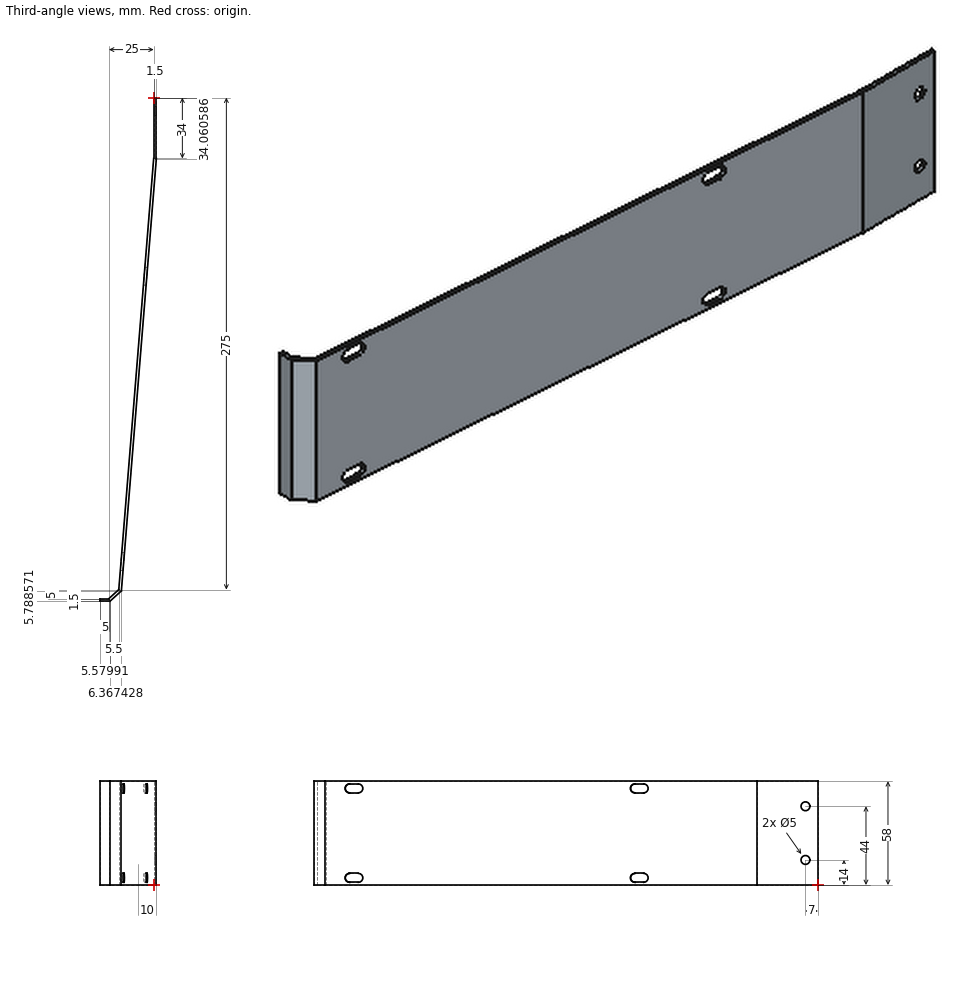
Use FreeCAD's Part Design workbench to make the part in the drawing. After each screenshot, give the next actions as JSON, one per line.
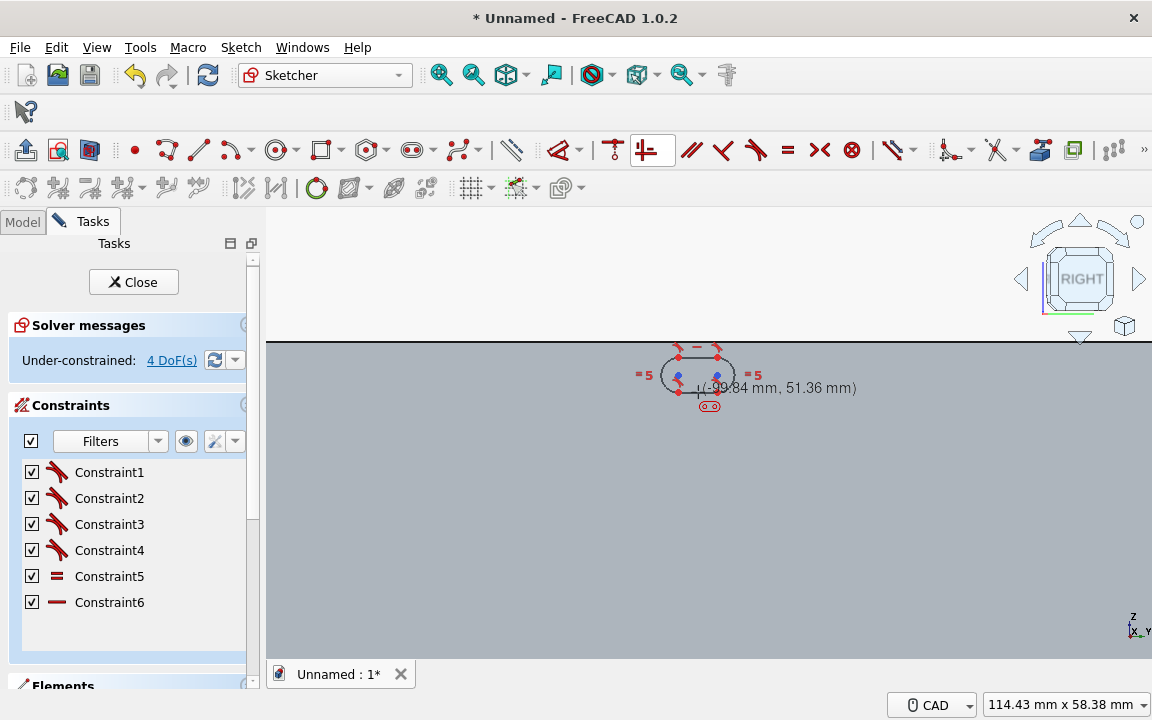
{"action": "scroll", "coordinate": [704, 388], "scroll_direction": "down", "scroll_amount": 7}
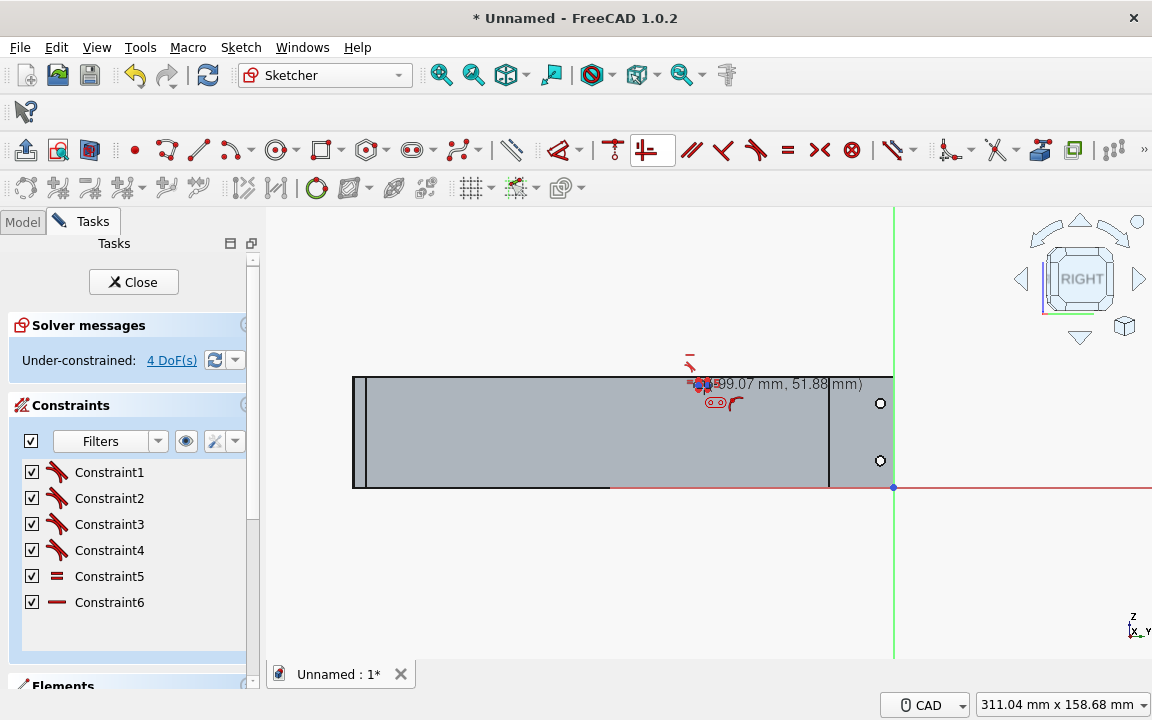
{"action": "scroll", "coordinate": [393, 385], "scroll_direction": "up", "scroll_amount": 8}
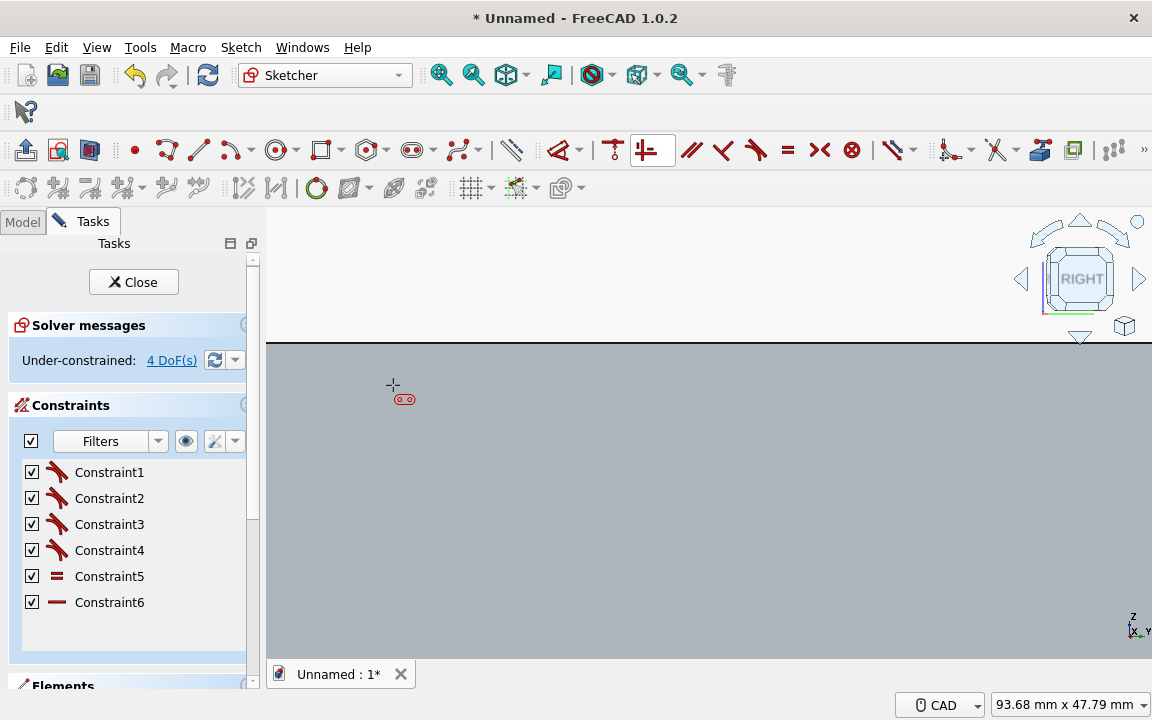
{"action": "scroll", "coordinate": [393, 385], "scroll_direction": "down", "scroll_amount": 8}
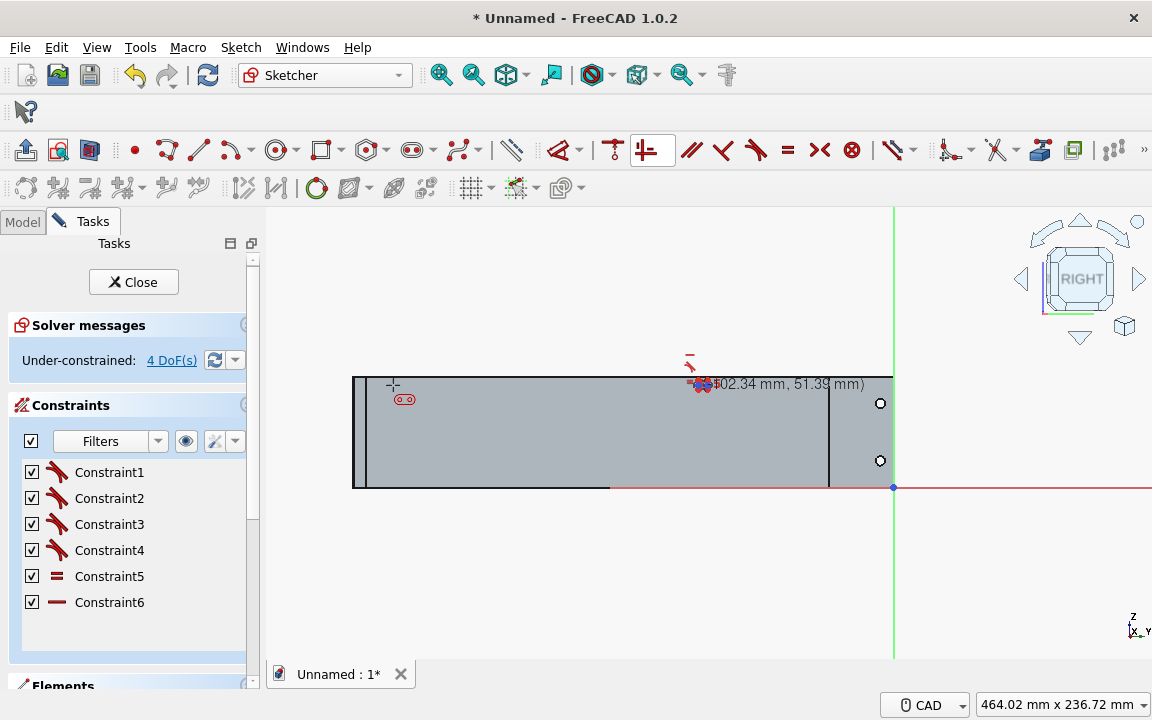
{"action": "left_click", "coordinate": [393, 385]}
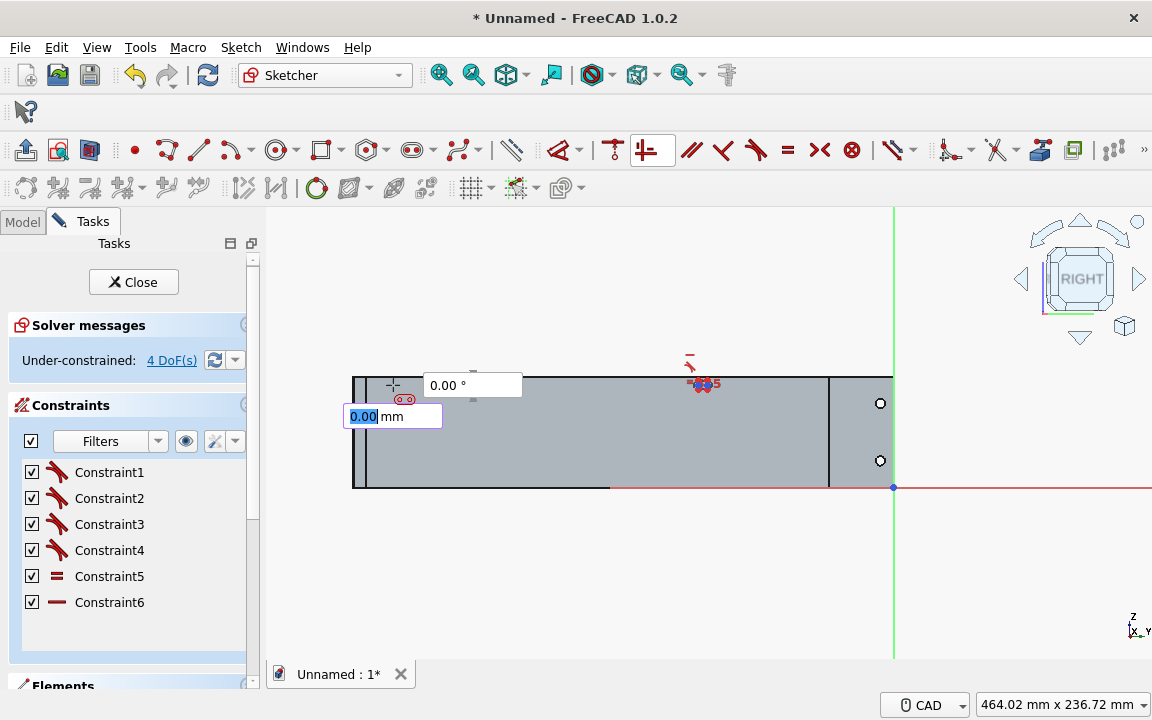
{"action": "scroll", "coordinate": [402, 385], "scroll_direction": "up", "scroll_amount": 3}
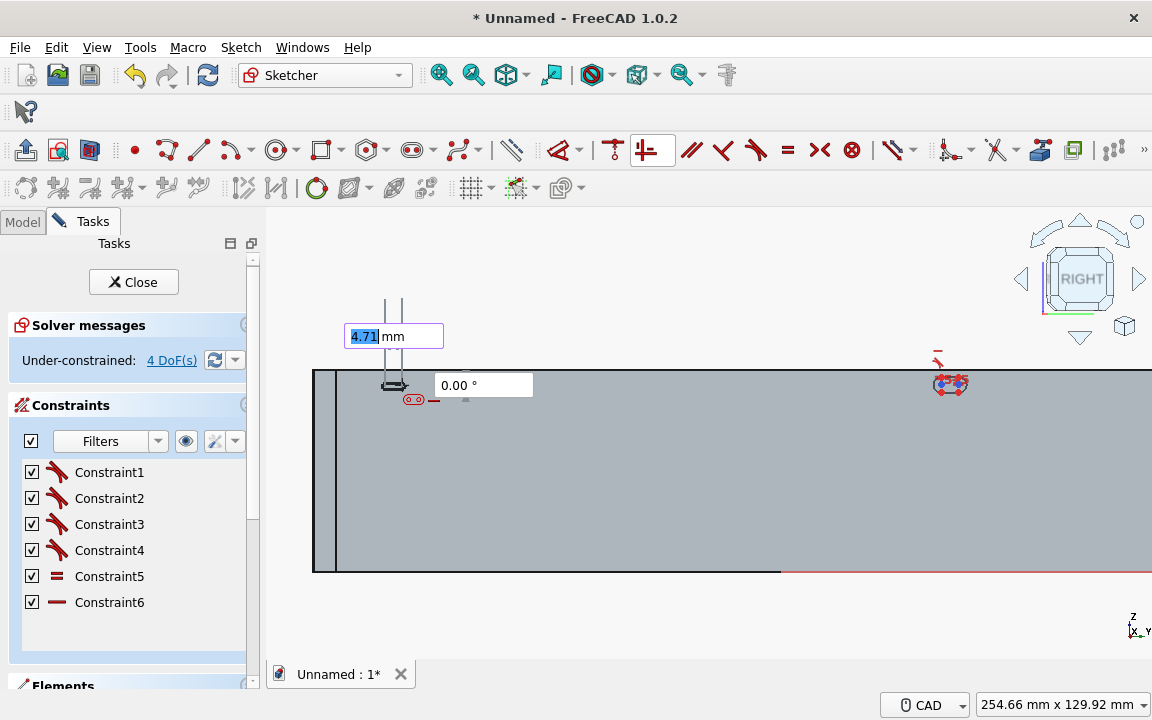
{"action": "left_click", "coordinate": [402, 385]}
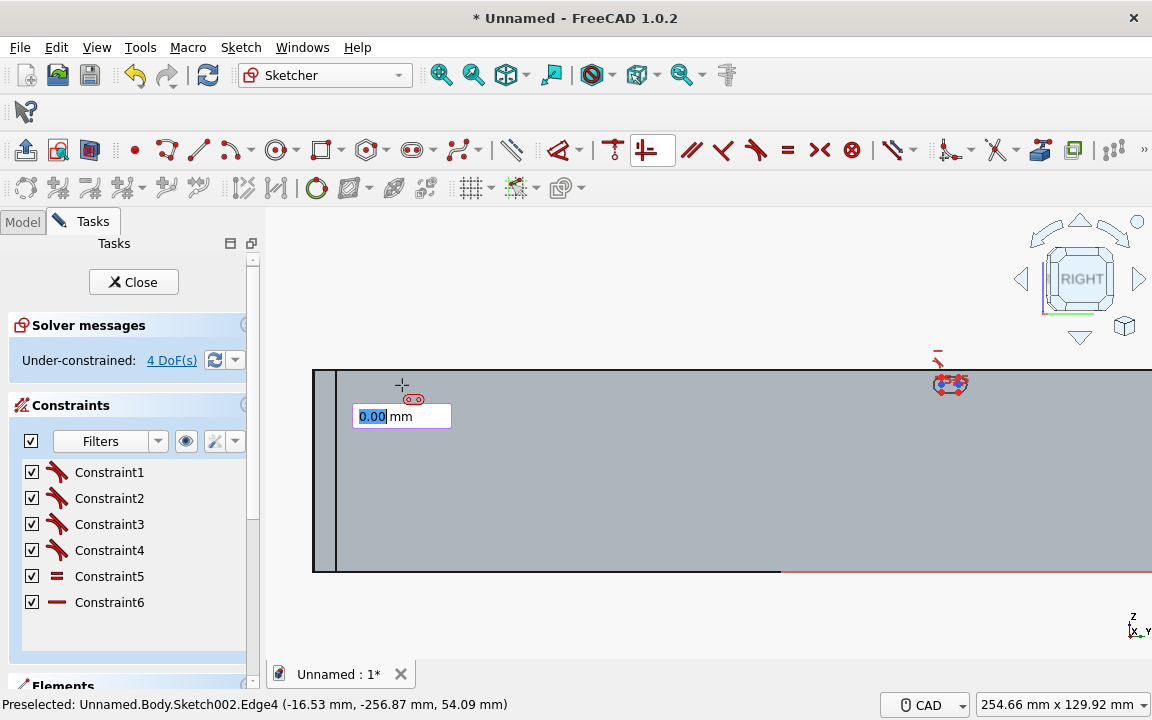
{"action": "scroll", "coordinate": [393, 392], "scroll_direction": "up", "scroll_amount": 4}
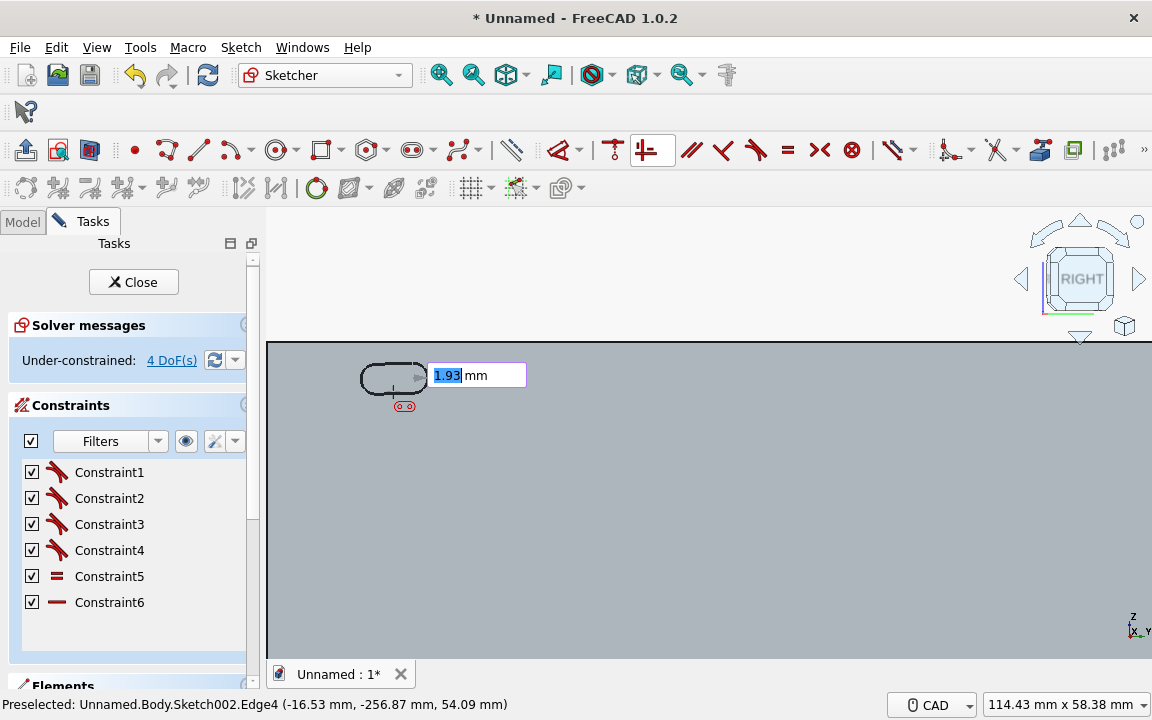
{"action": "left_click", "coordinate": [394, 393]}
{"action": "key", "text": "Escape"}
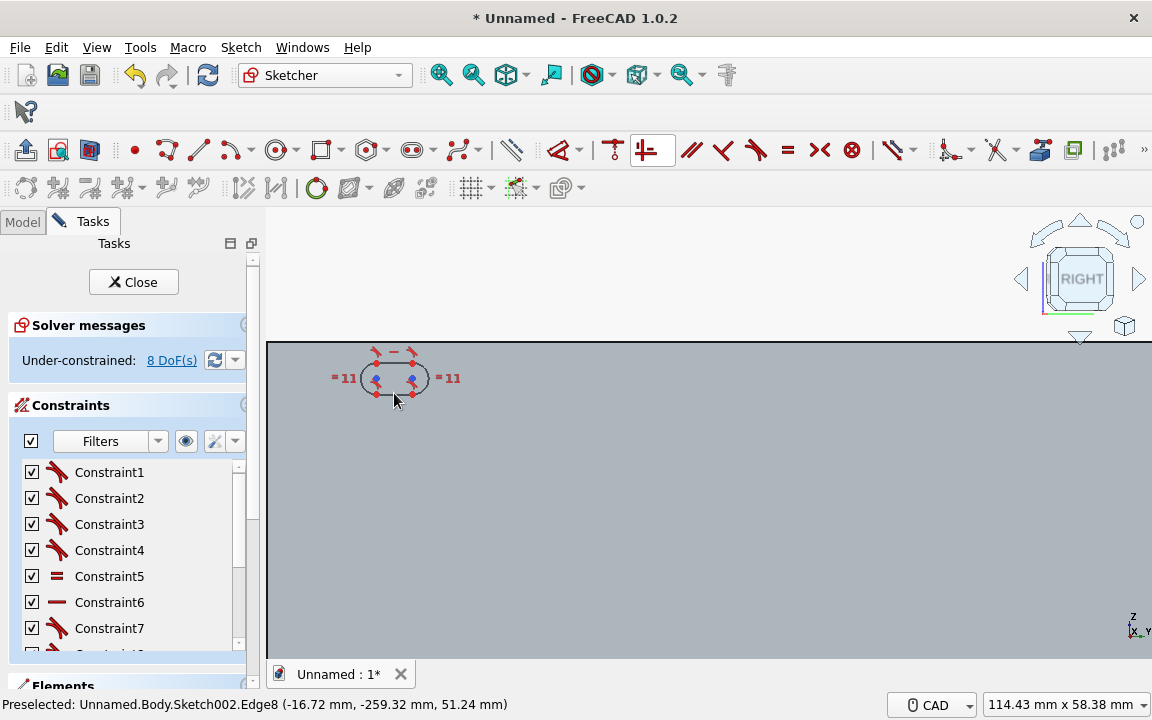
{"action": "scroll", "coordinate": [398, 387], "scroll_direction": "down", "scroll_amount": 7}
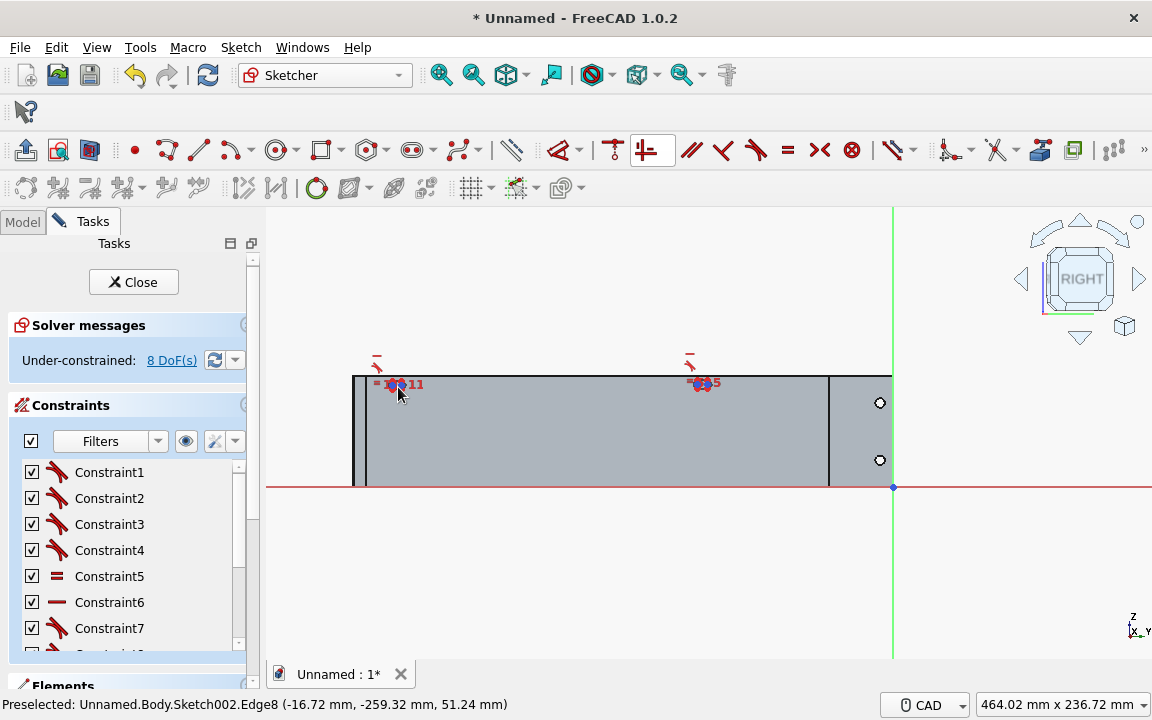
{"action": "scroll", "coordinate": [694, 382], "scroll_direction": "up", "scroll_amount": 7}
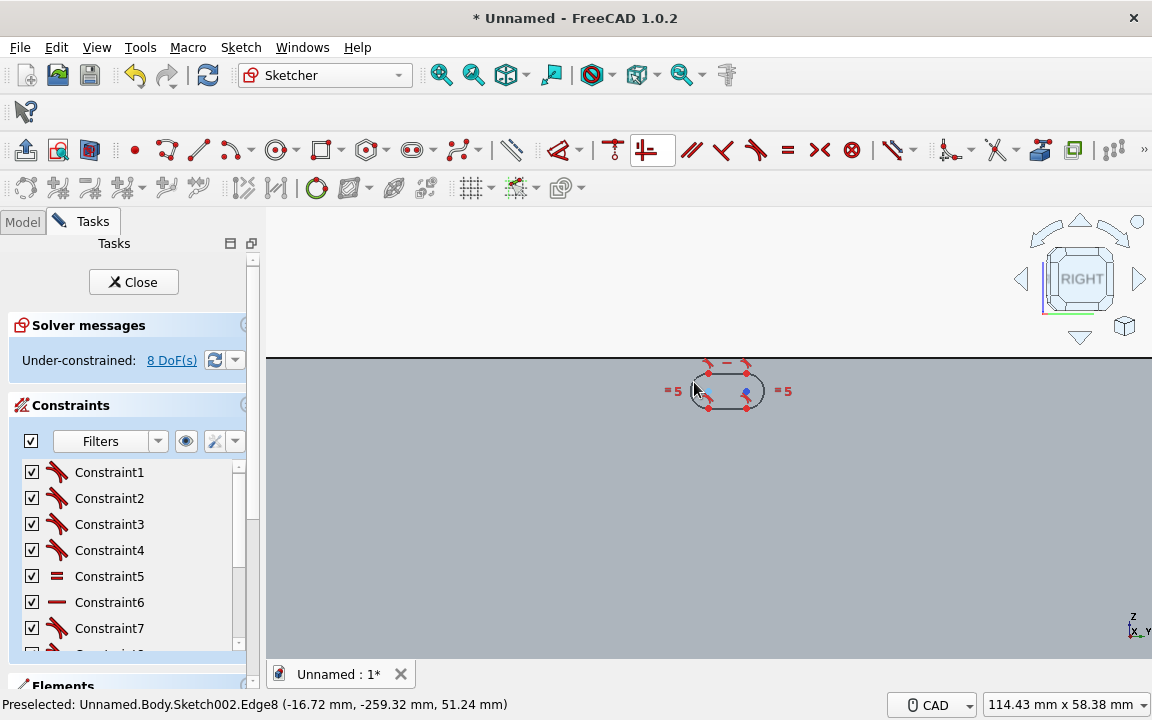
{"action": "left_click", "coordinate": [694, 381]}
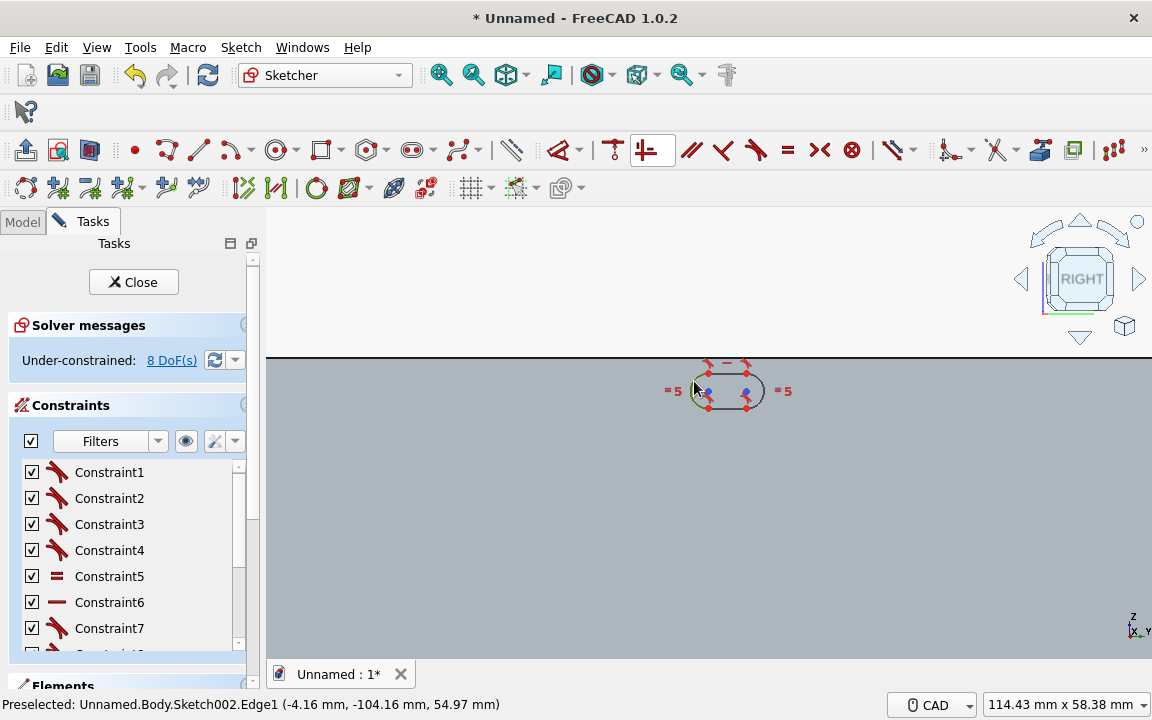
{"action": "scroll", "coordinate": [695, 382], "scroll_direction": "down", "scroll_amount": 7}